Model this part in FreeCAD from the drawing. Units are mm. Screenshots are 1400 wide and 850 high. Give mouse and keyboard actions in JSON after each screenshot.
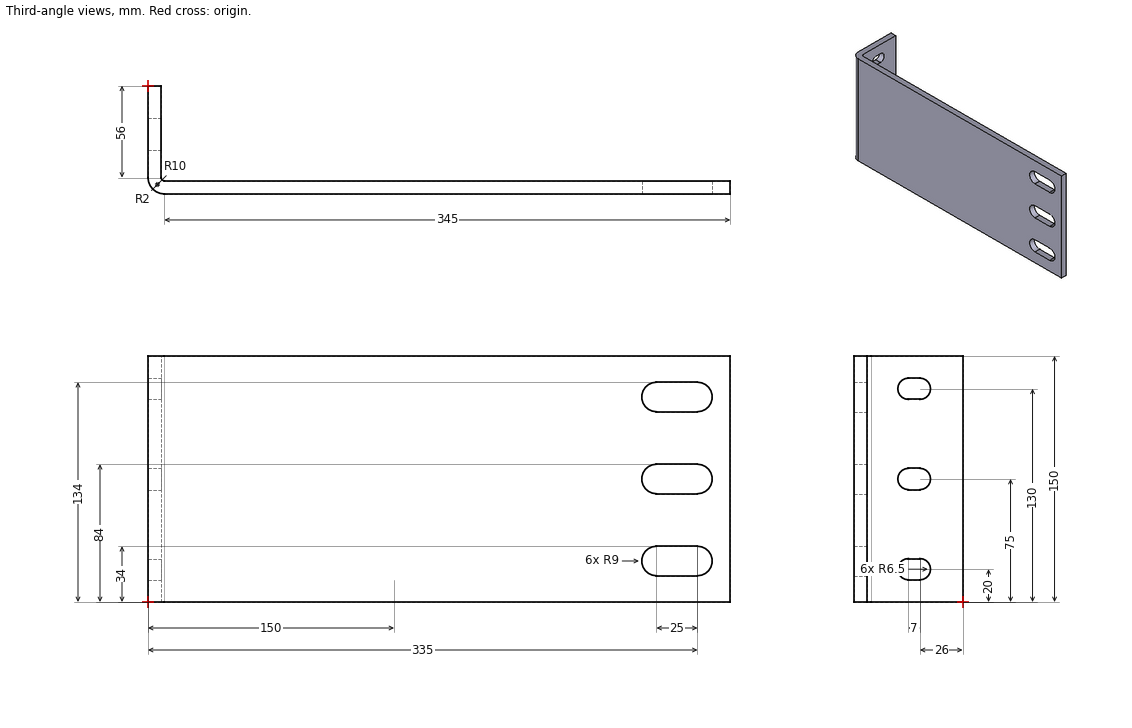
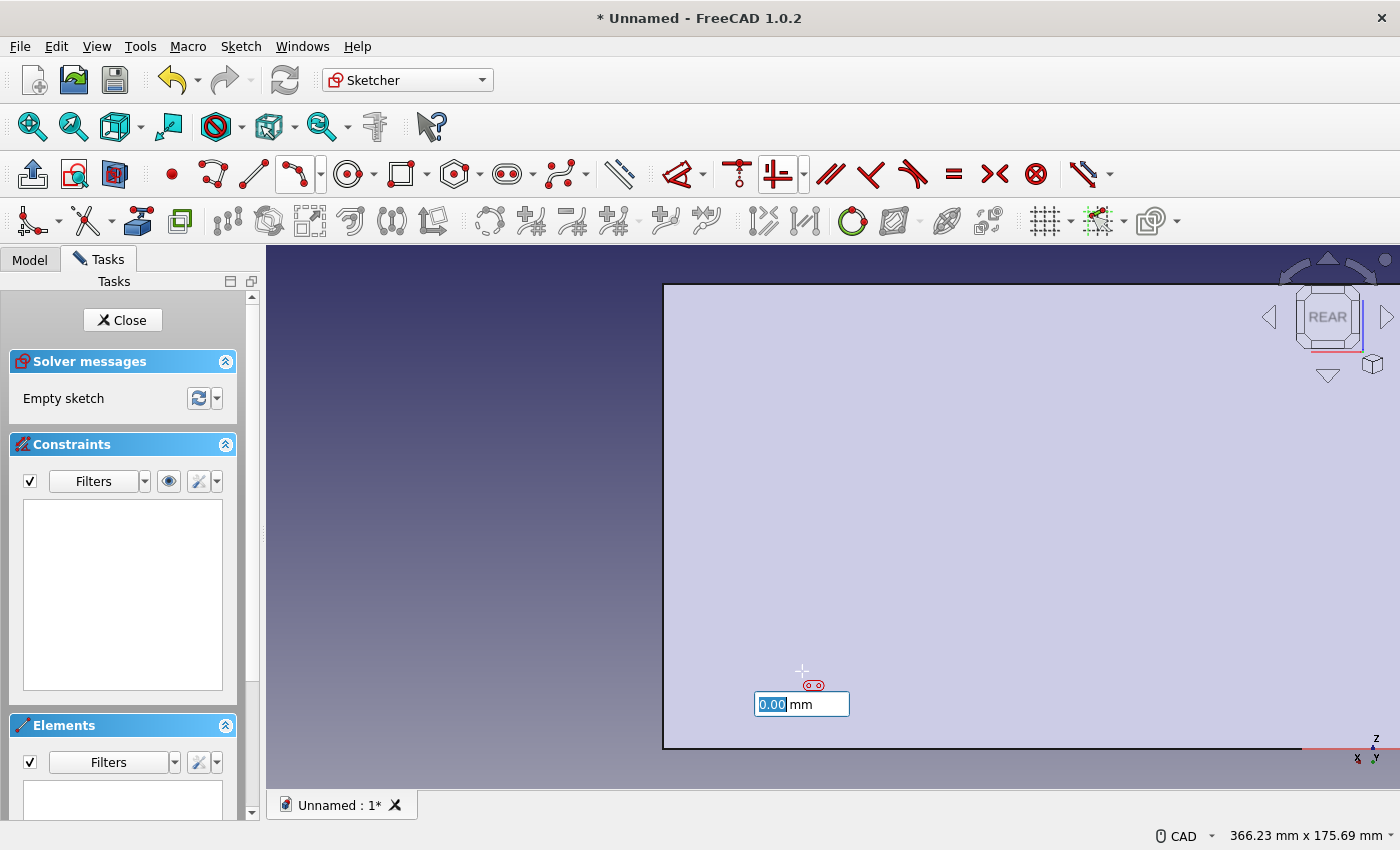
{"action": "left_click", "coordinate": [764, 699]}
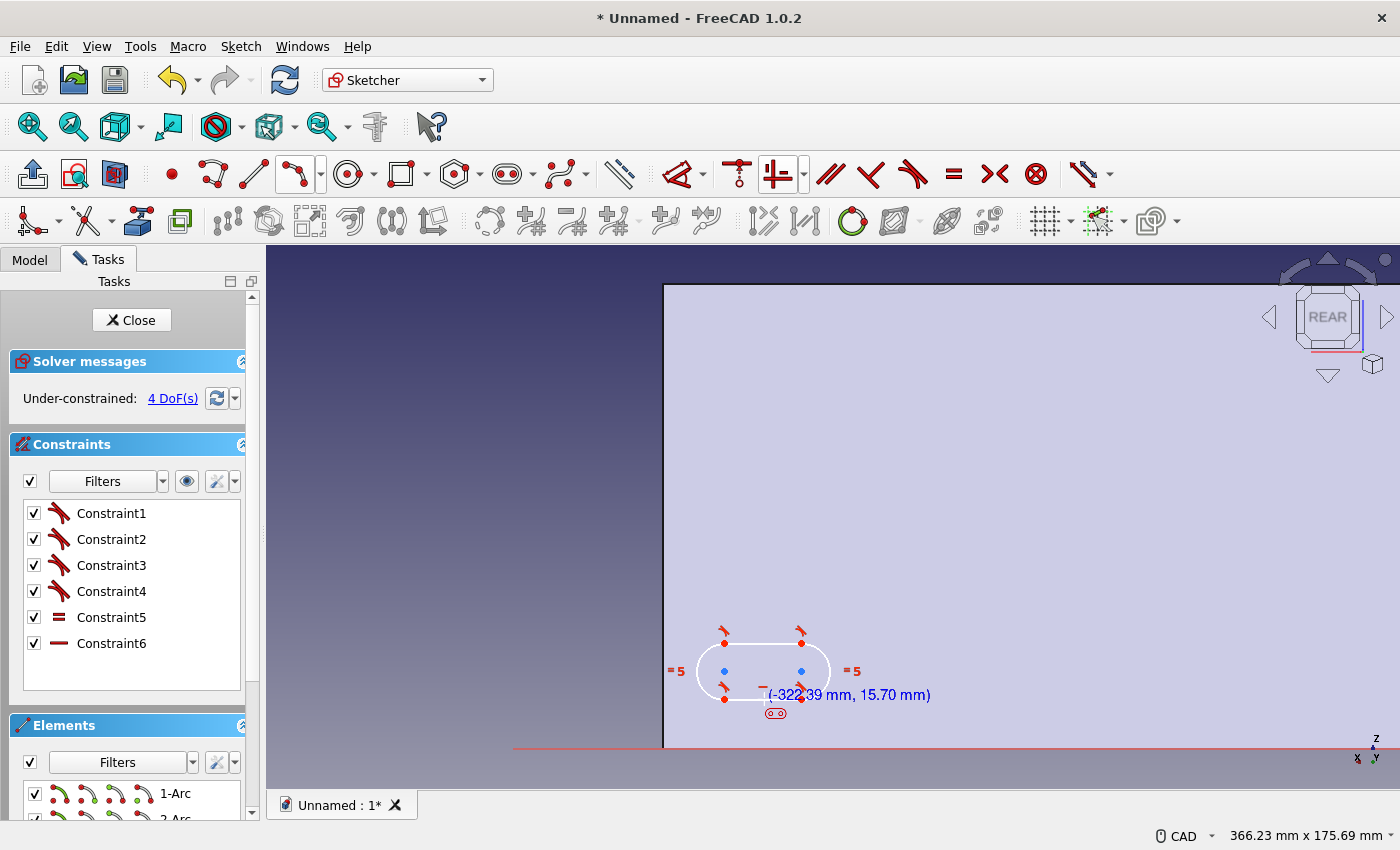
{"action": "left_click", "coordinate": [725, 516]}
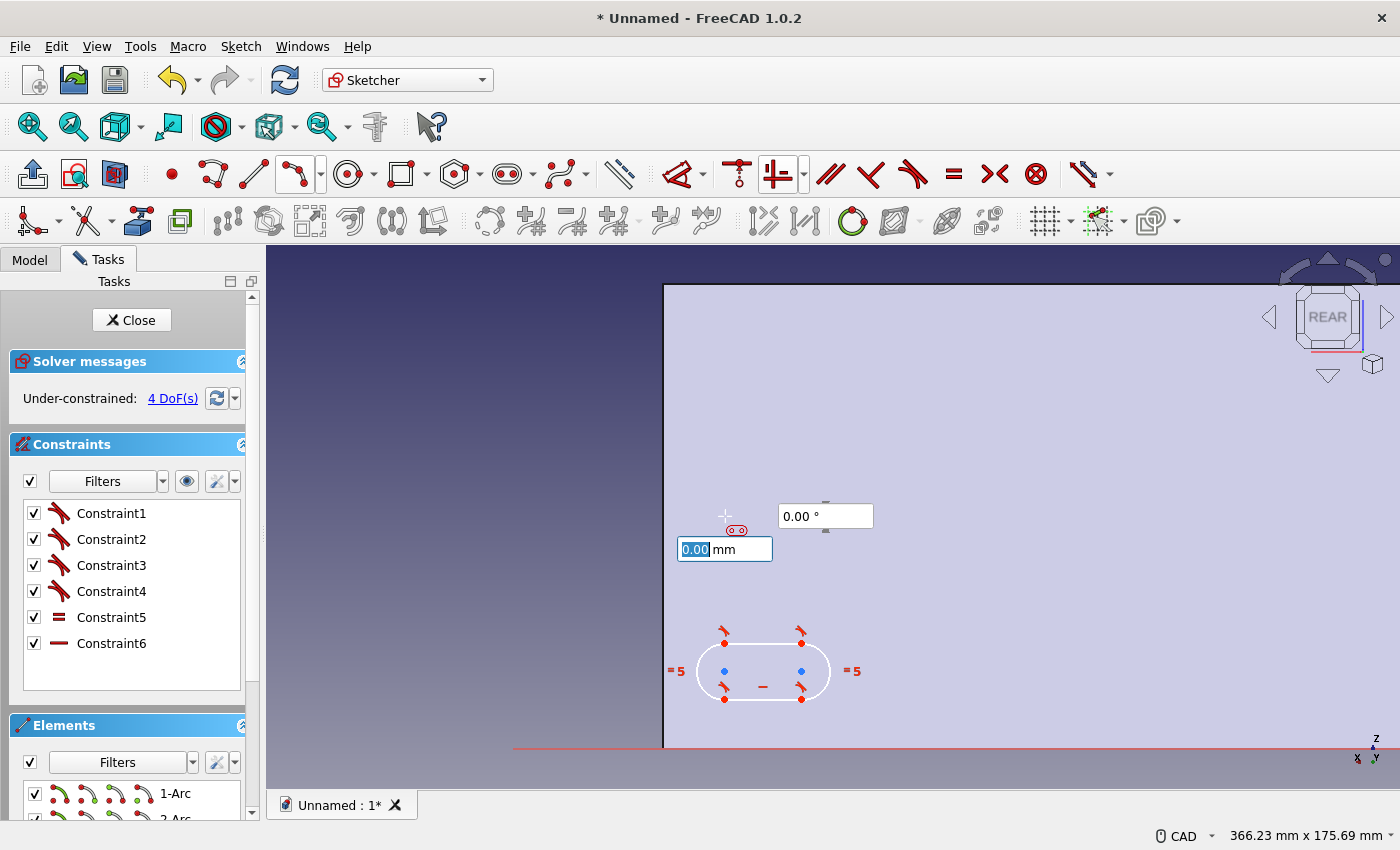
{"action": "left_click", "coordinate": [802, 516]}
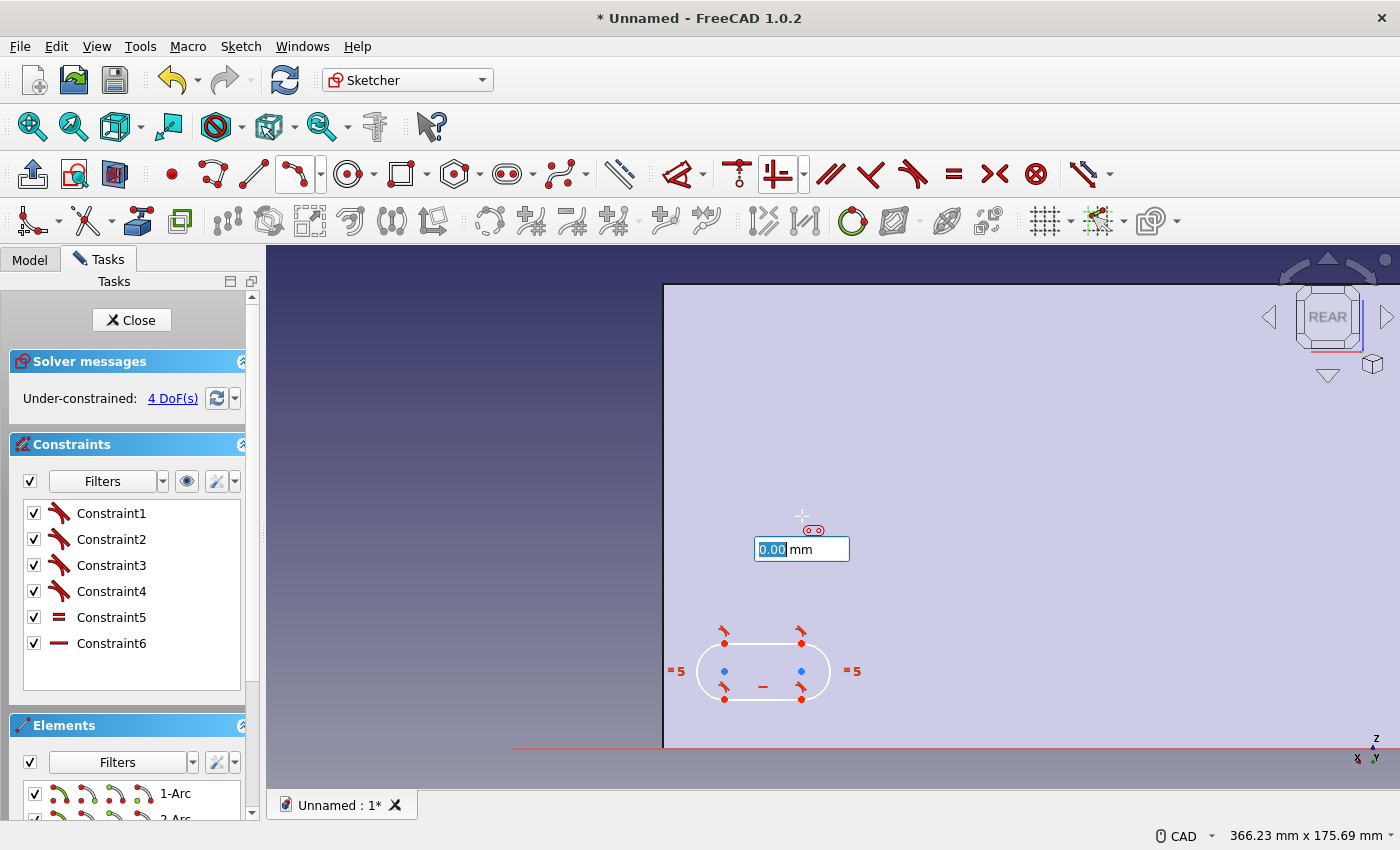
{"action": "left_click", "coordinate": [764, 544]}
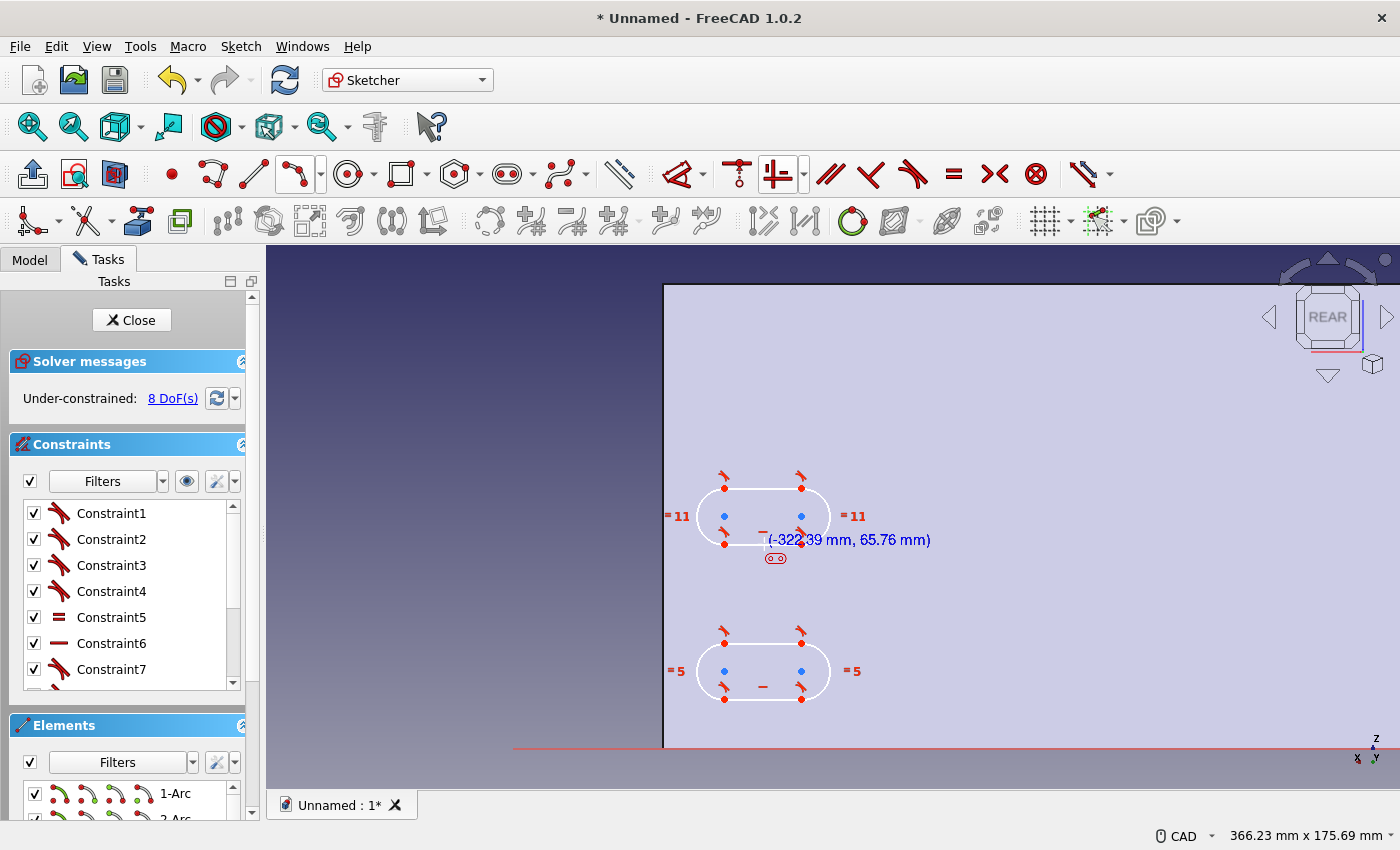
{"action": "left_click", "coordinate": [725, 362]}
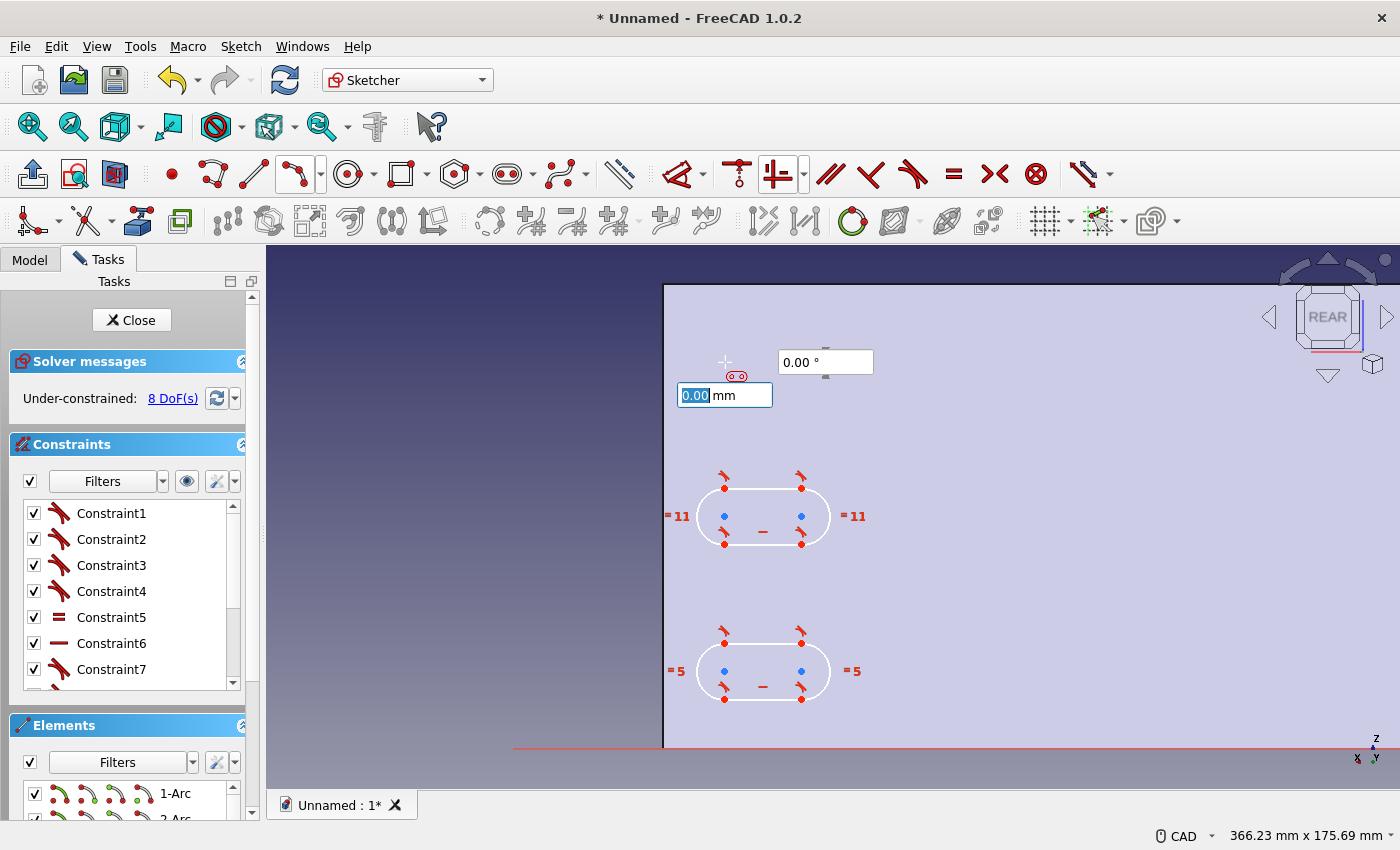
{"action": "left_click", "coordinate": [802, 362]}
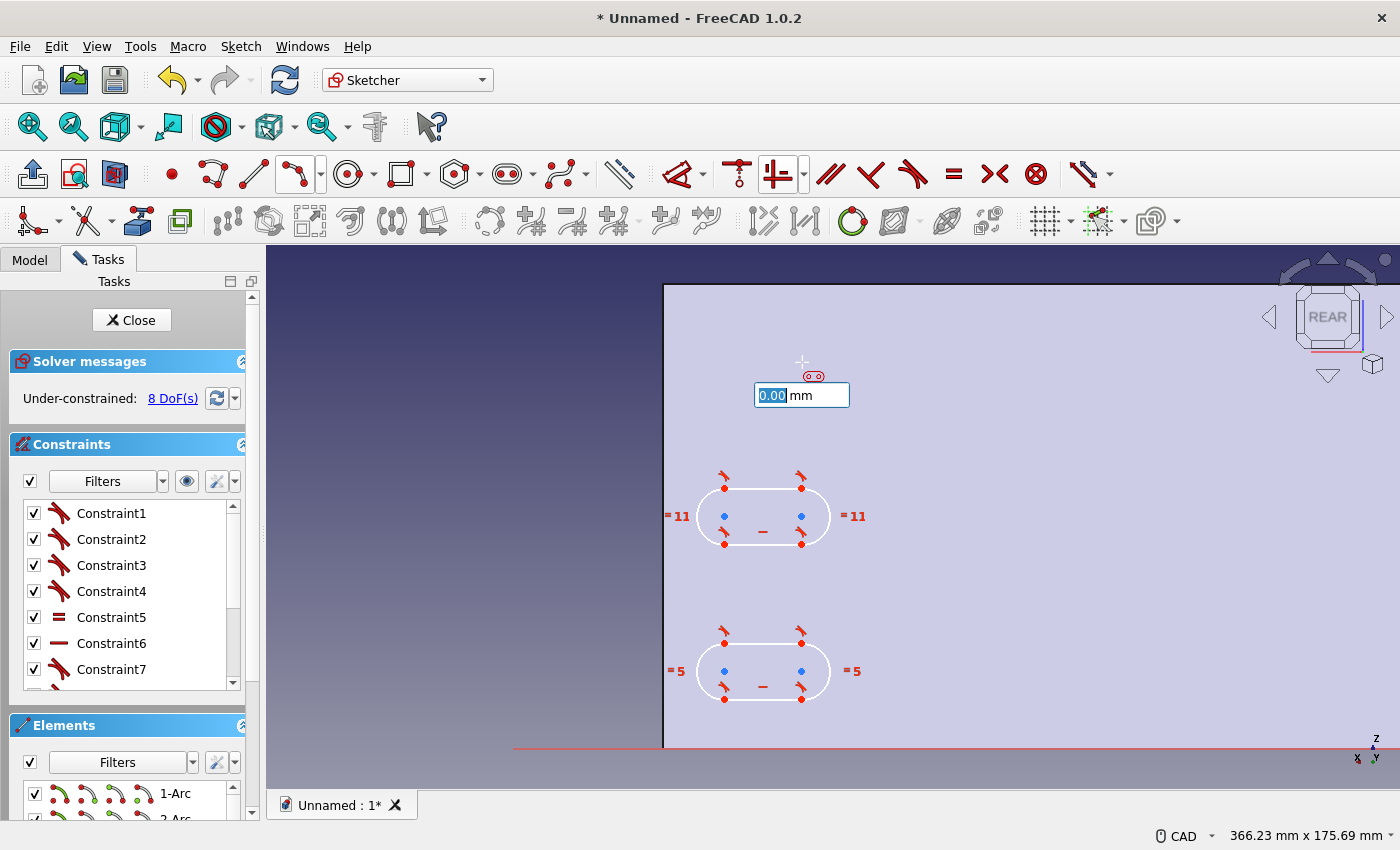
{"action": "left_click", "coordinate": [764, 389]}
{"action": "key", "text": "Escape"}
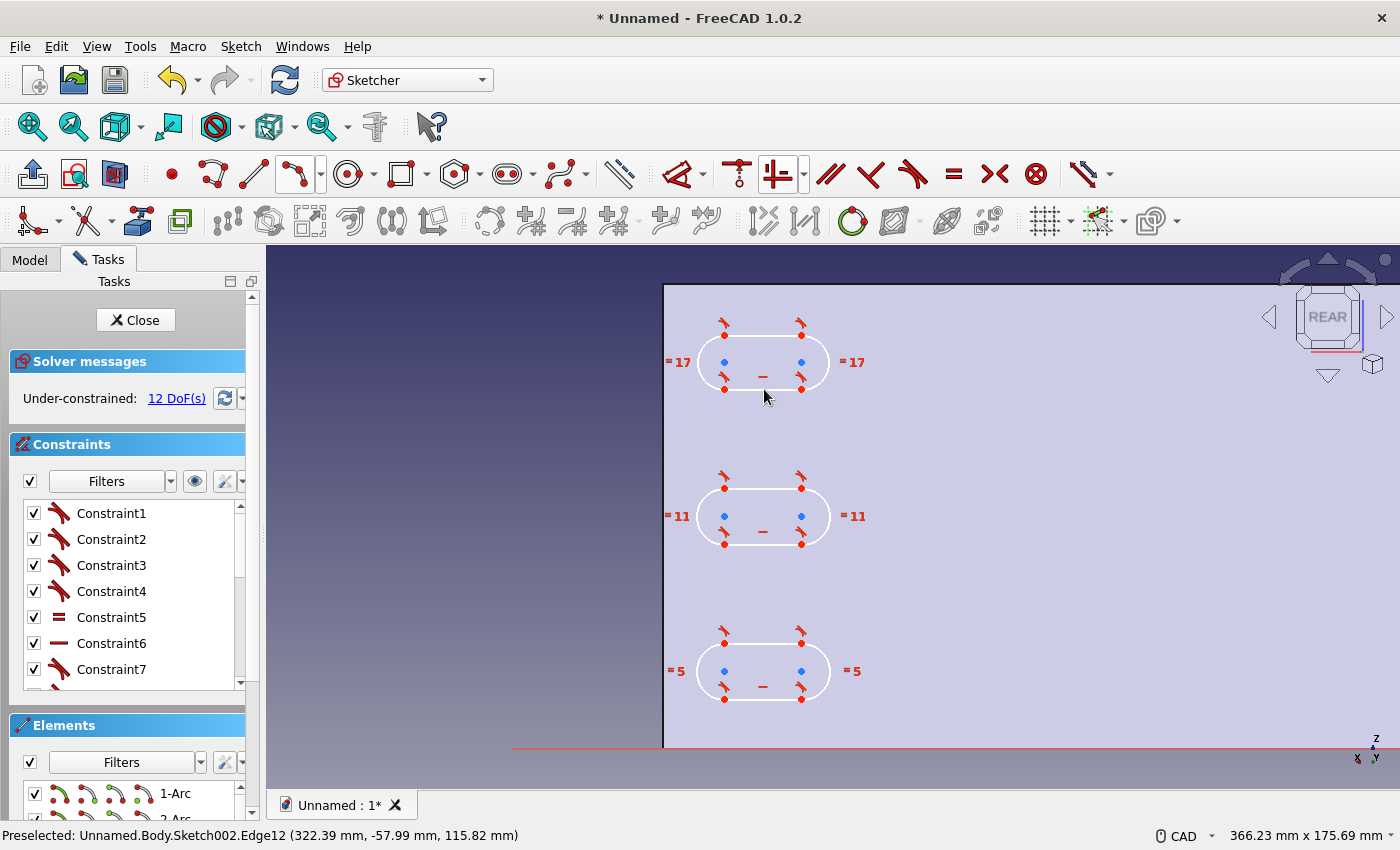
{"action": "left_click", "coordinate": [702, 656]}